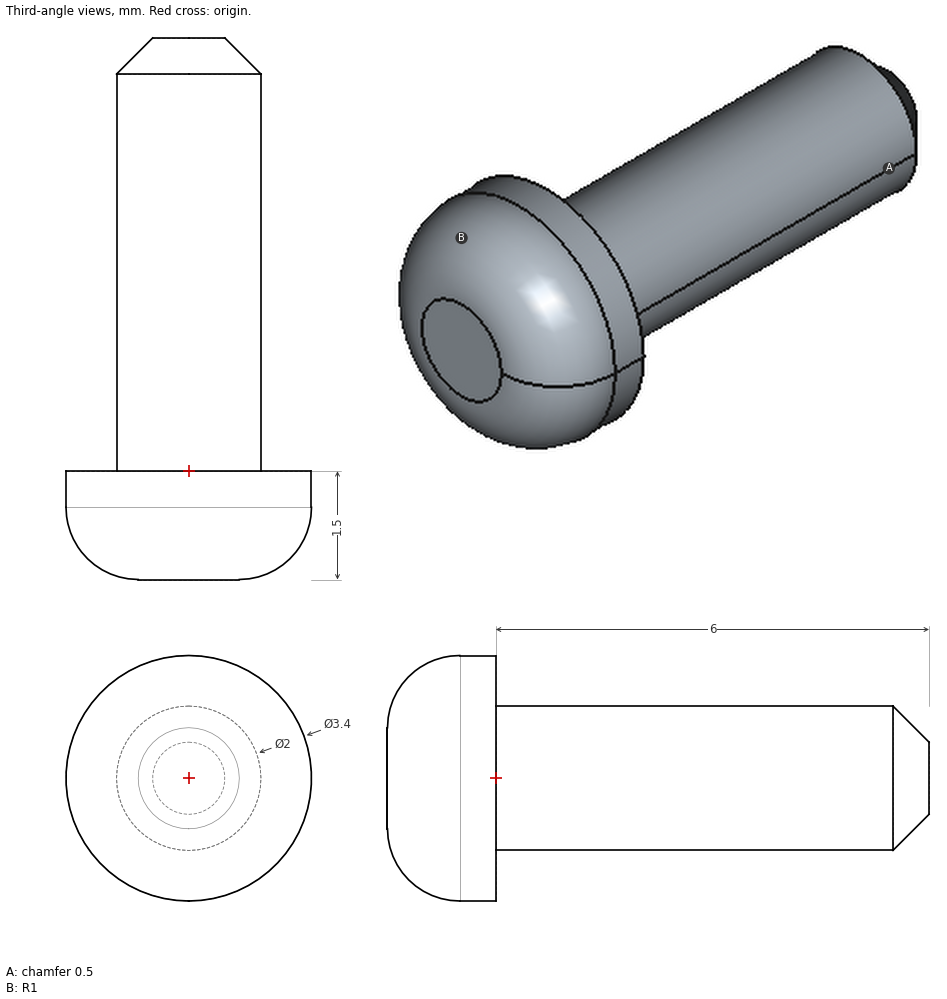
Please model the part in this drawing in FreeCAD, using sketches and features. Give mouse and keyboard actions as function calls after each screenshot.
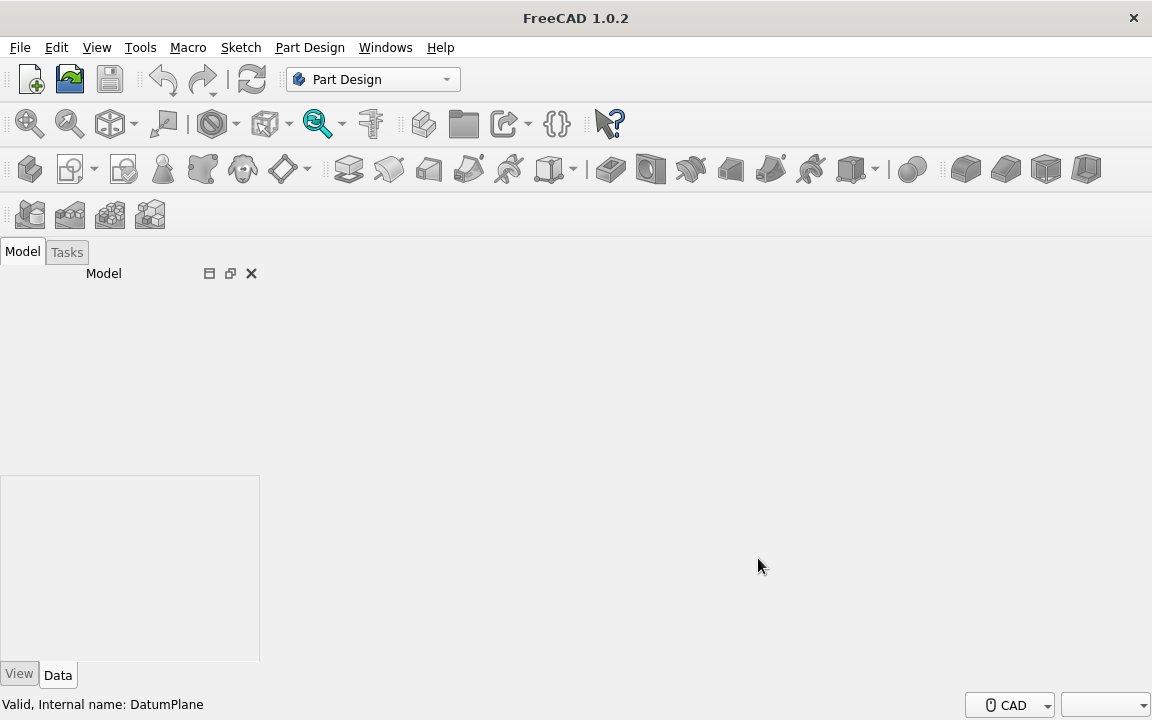
click(30, 80)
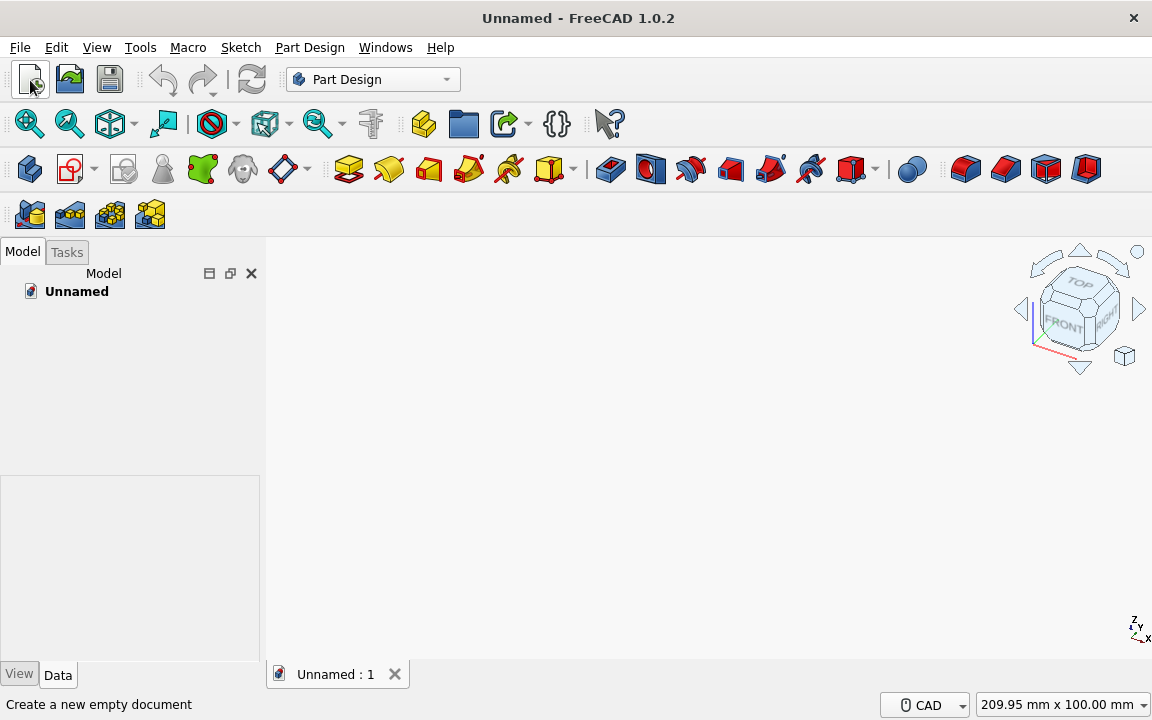
click(70, 170)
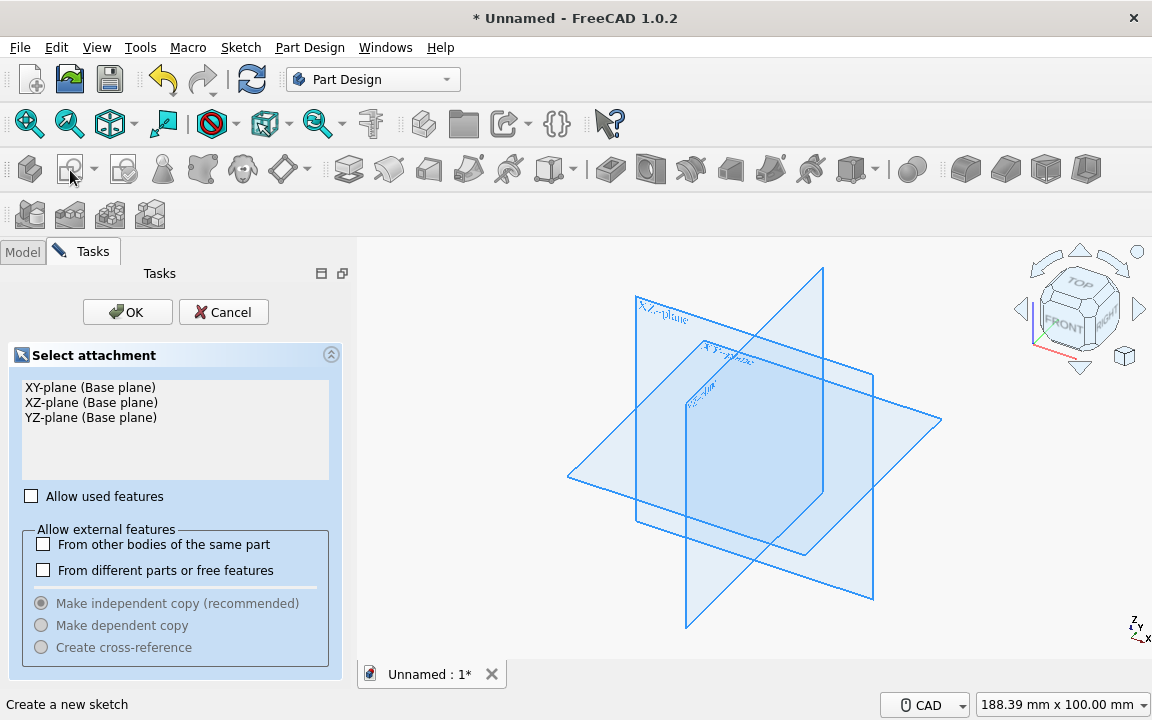
click(82, 402)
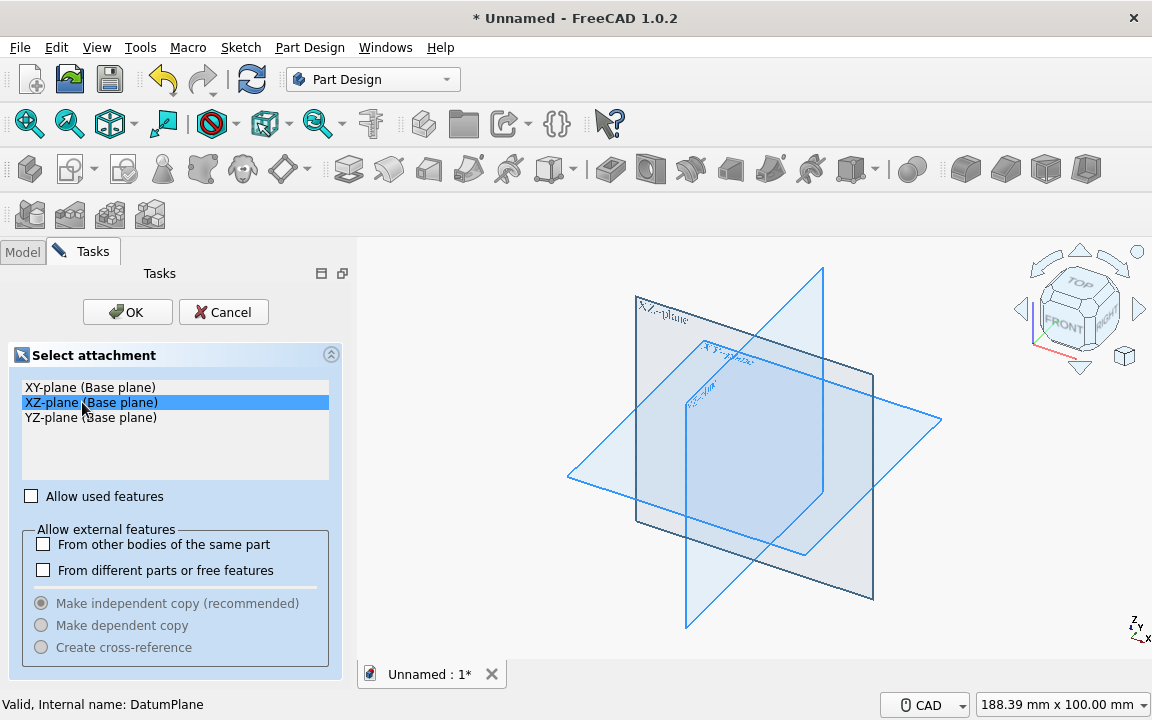
click(128, 312)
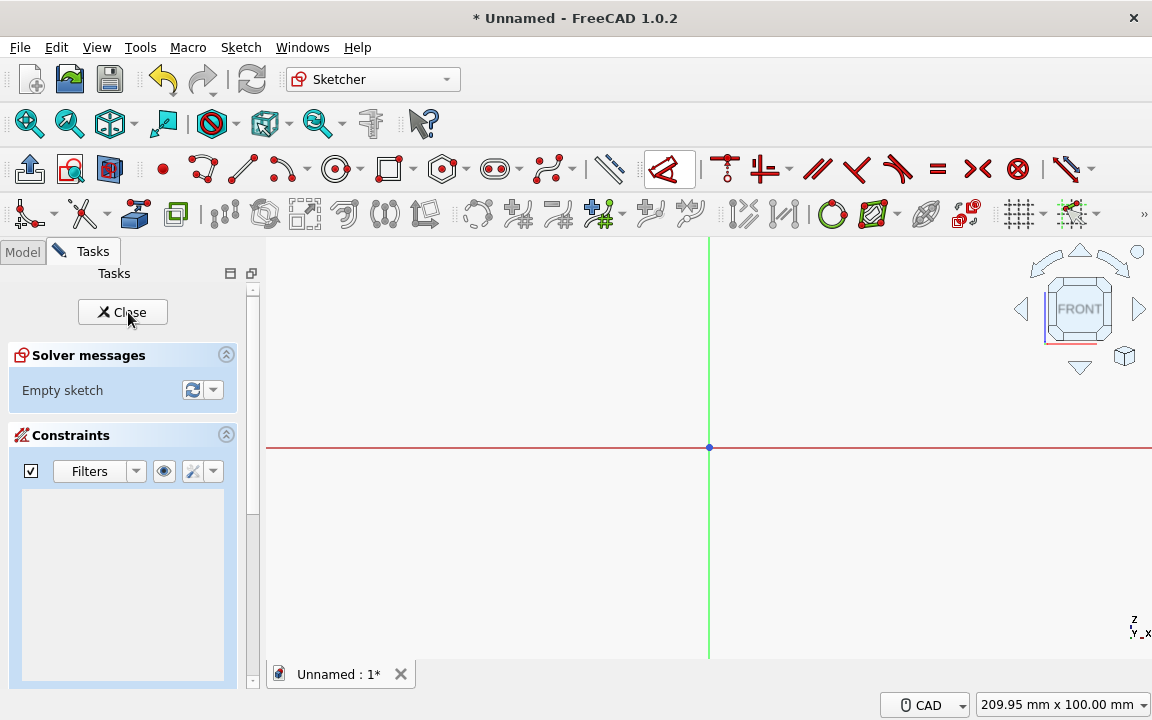
scroll(713, 448, up, 15)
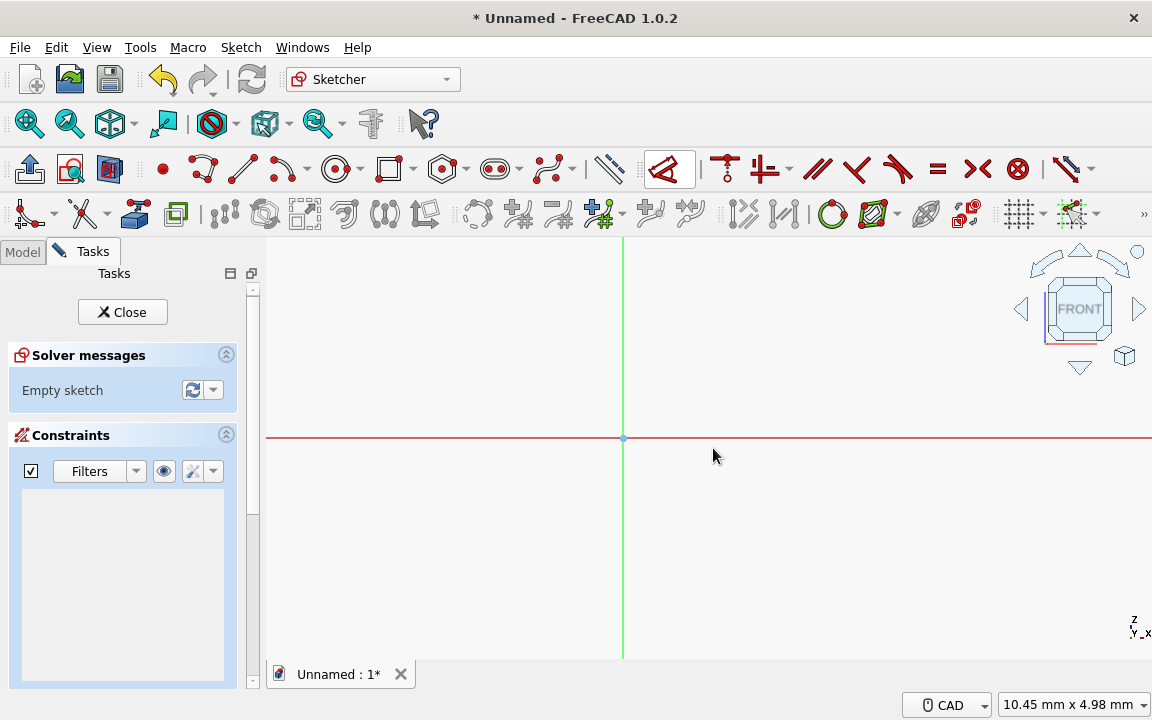
scroll(587, 419, up, 2)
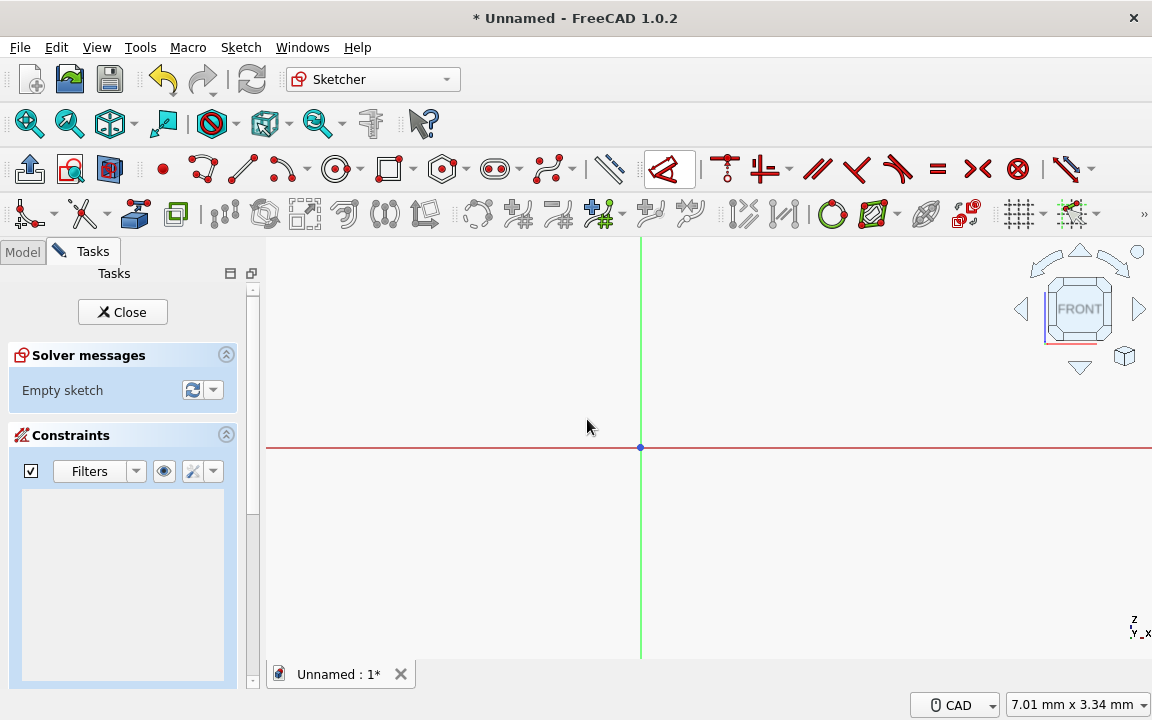
click(336, 170)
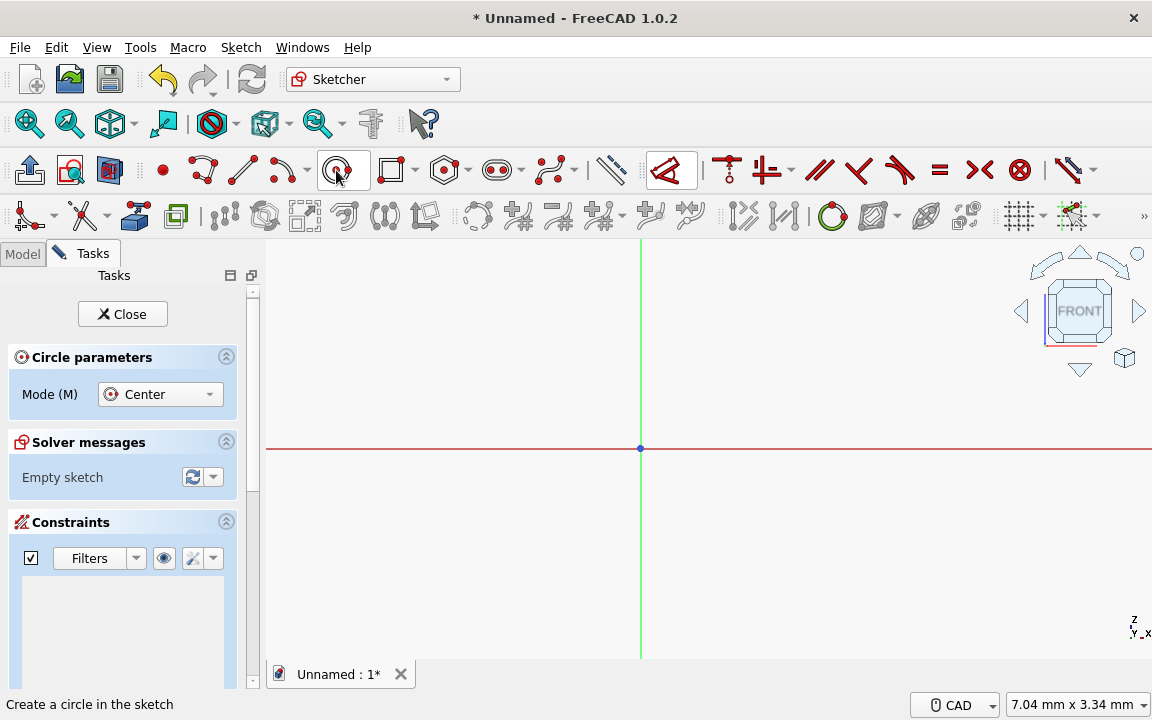
click(641, 449)
move(730, 360)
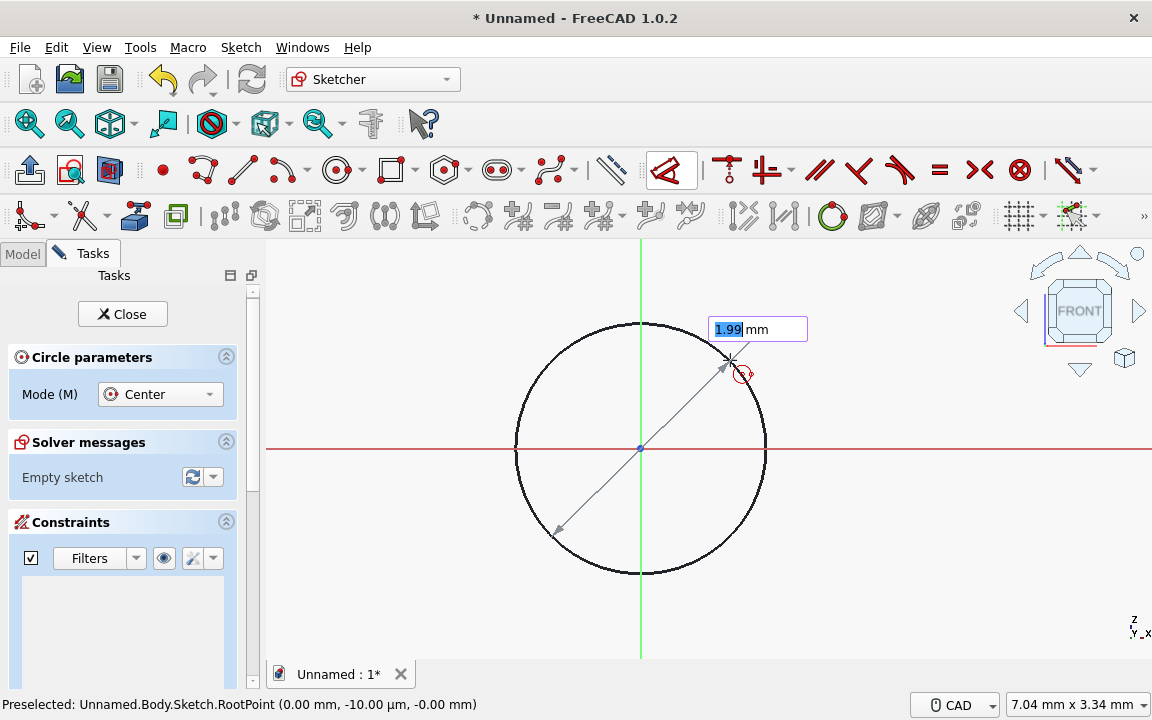
text(2)
key(Return)
key(Escape)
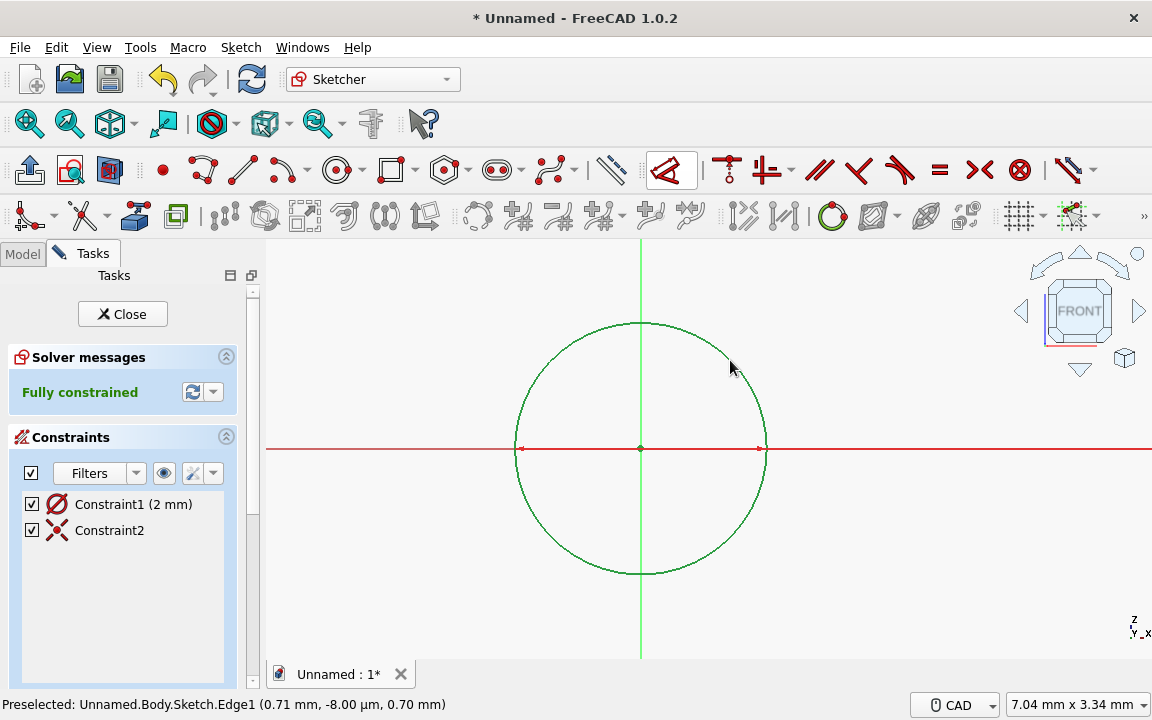
click(123, 314)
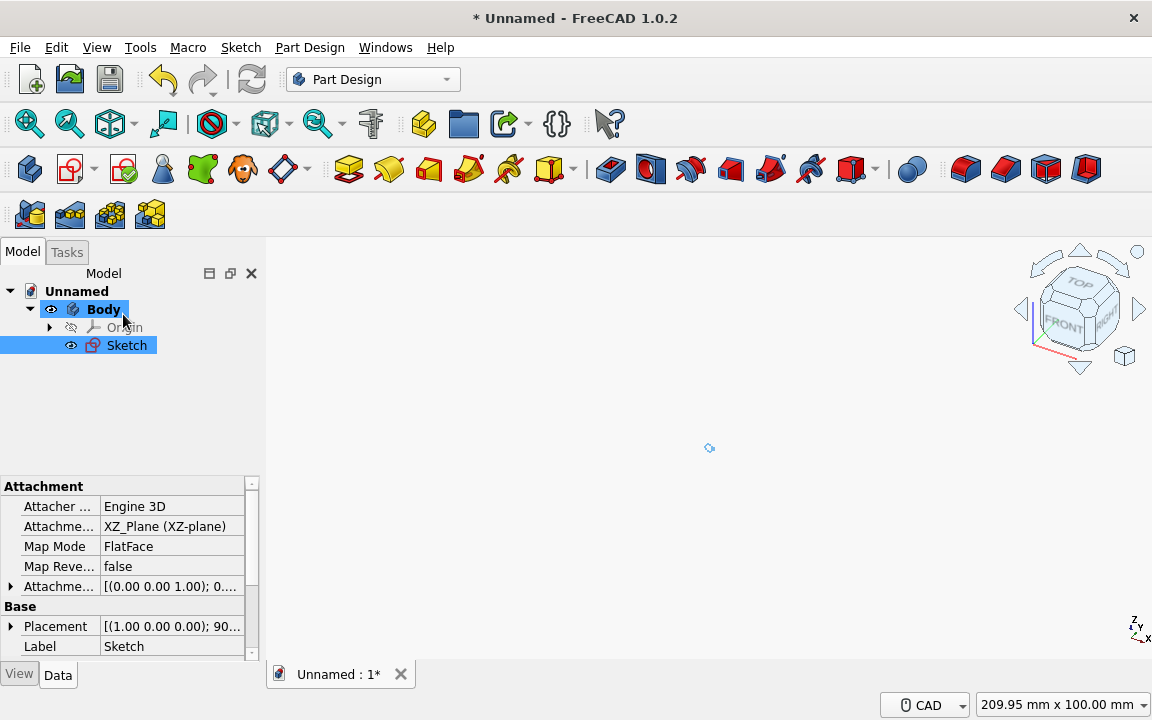
click(350, 170)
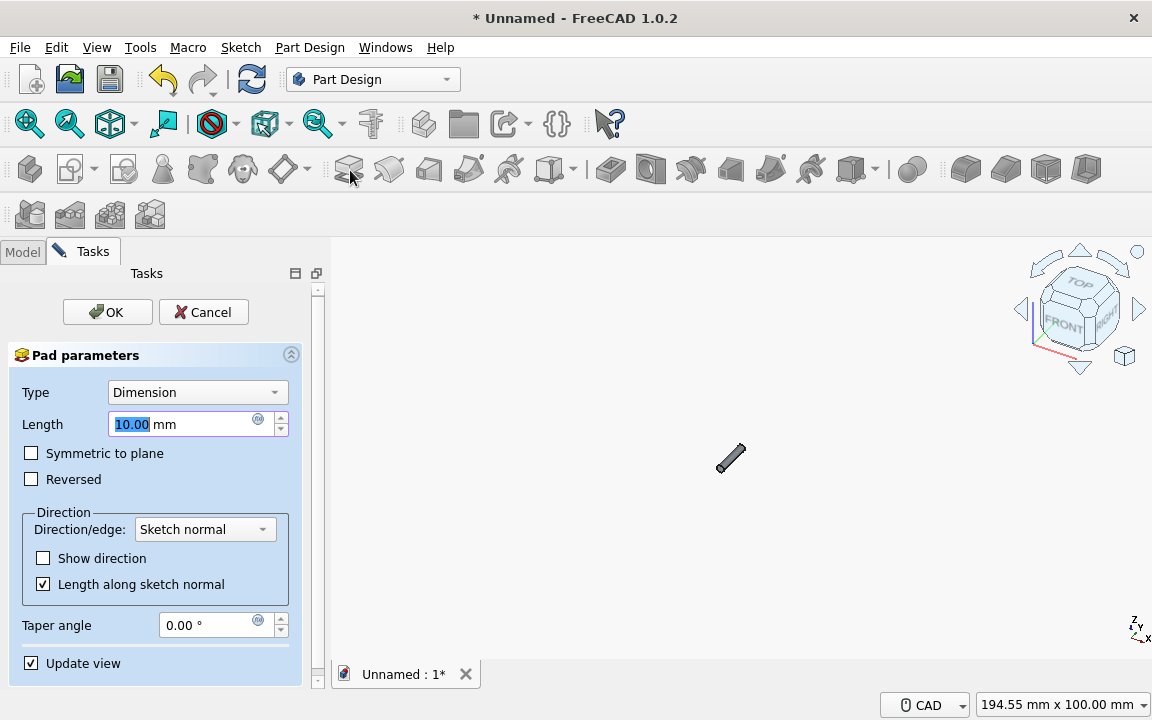
text(6)
key(Tab)